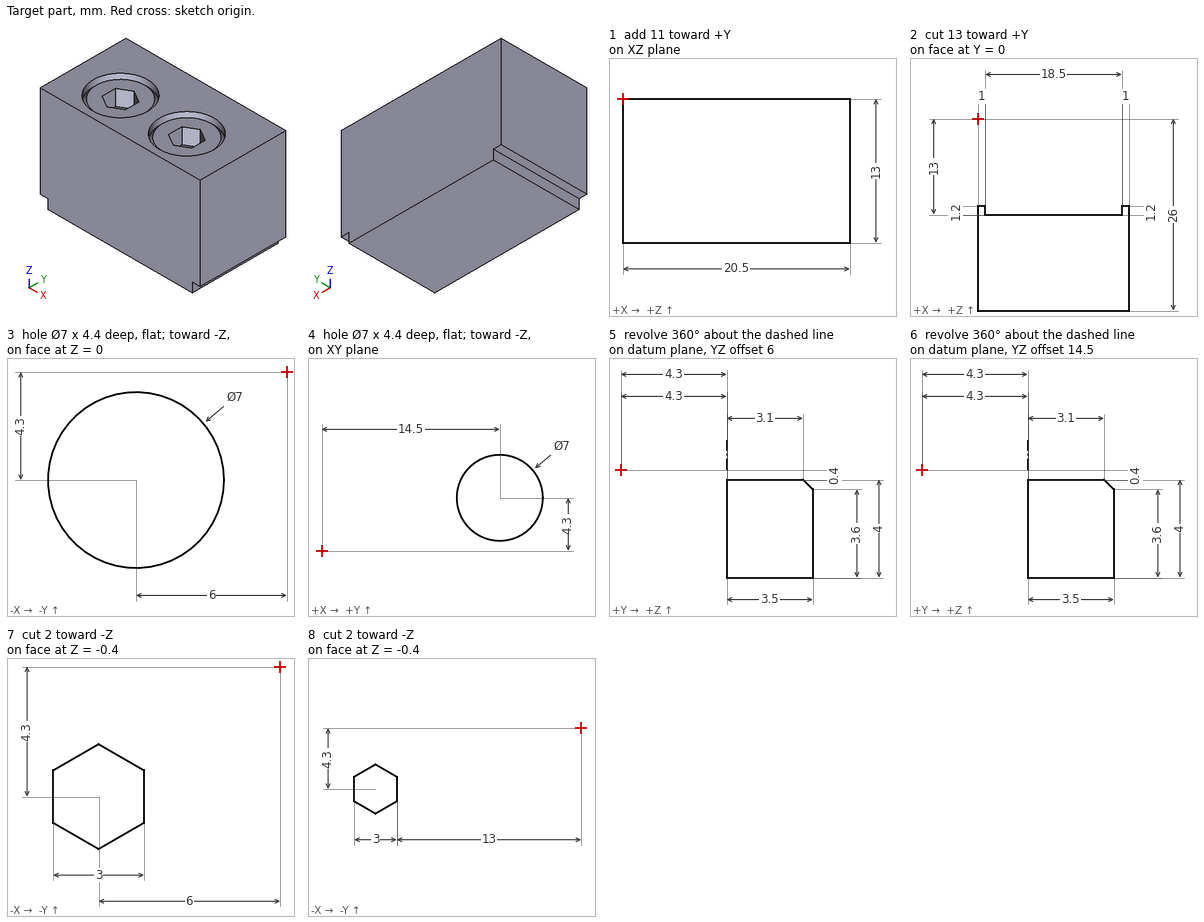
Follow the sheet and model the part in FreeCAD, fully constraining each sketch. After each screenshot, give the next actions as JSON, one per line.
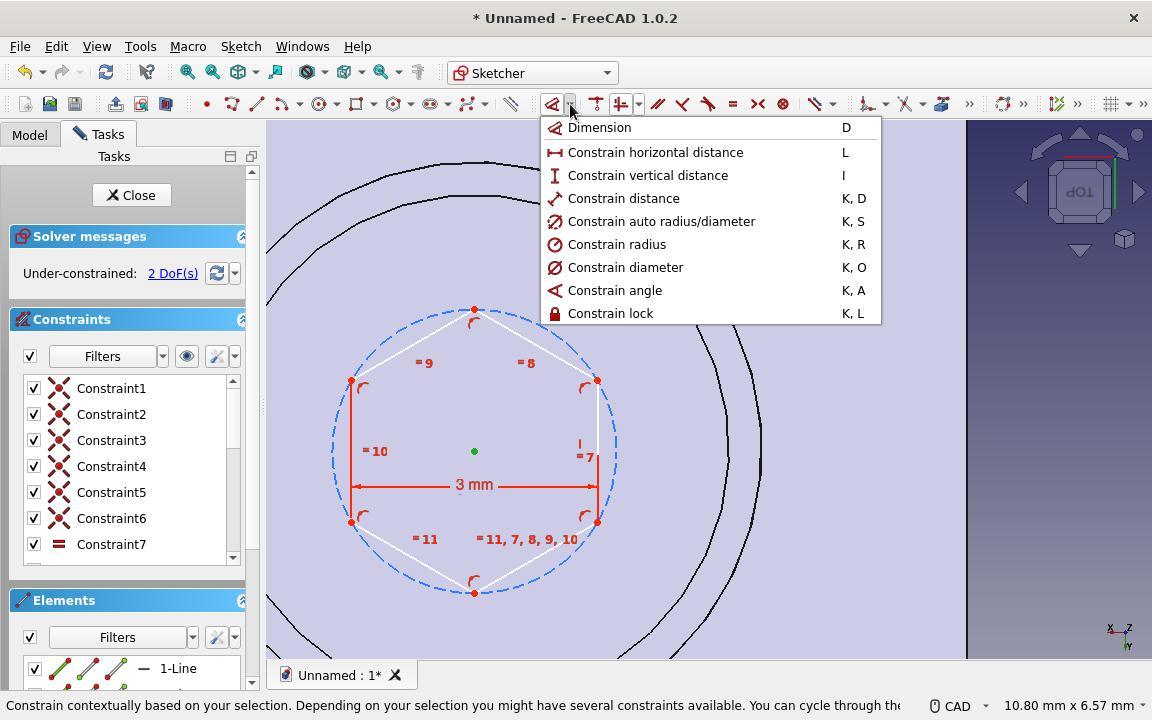
{"action": "left_click", "coordinate": [711, 152]}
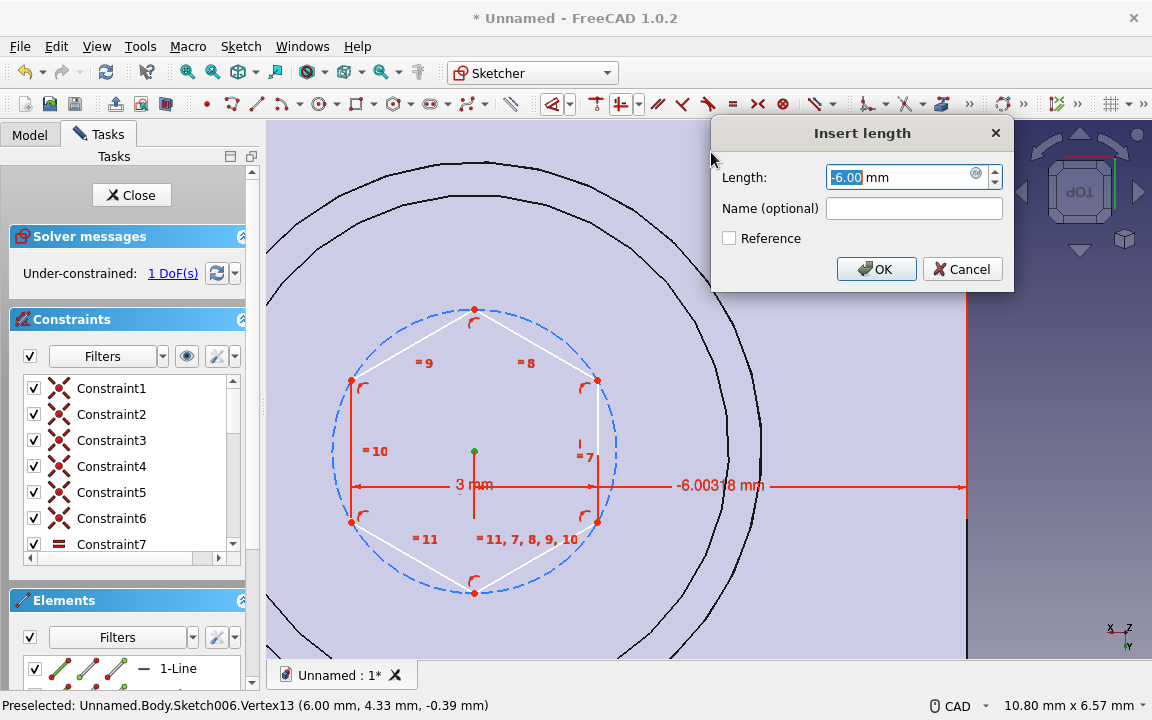
{"action": "type", "text": "-6"}
{"action": "key", "text": "Return"}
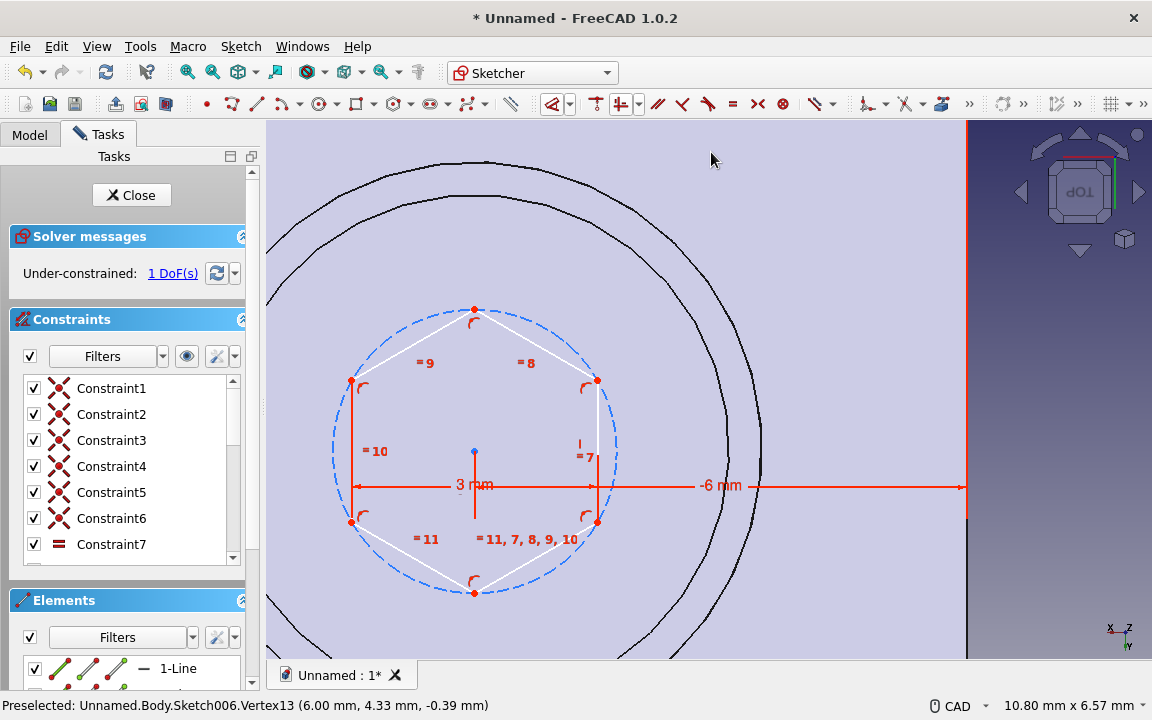
{"action": "left_click", "coordinate": [475, 451]}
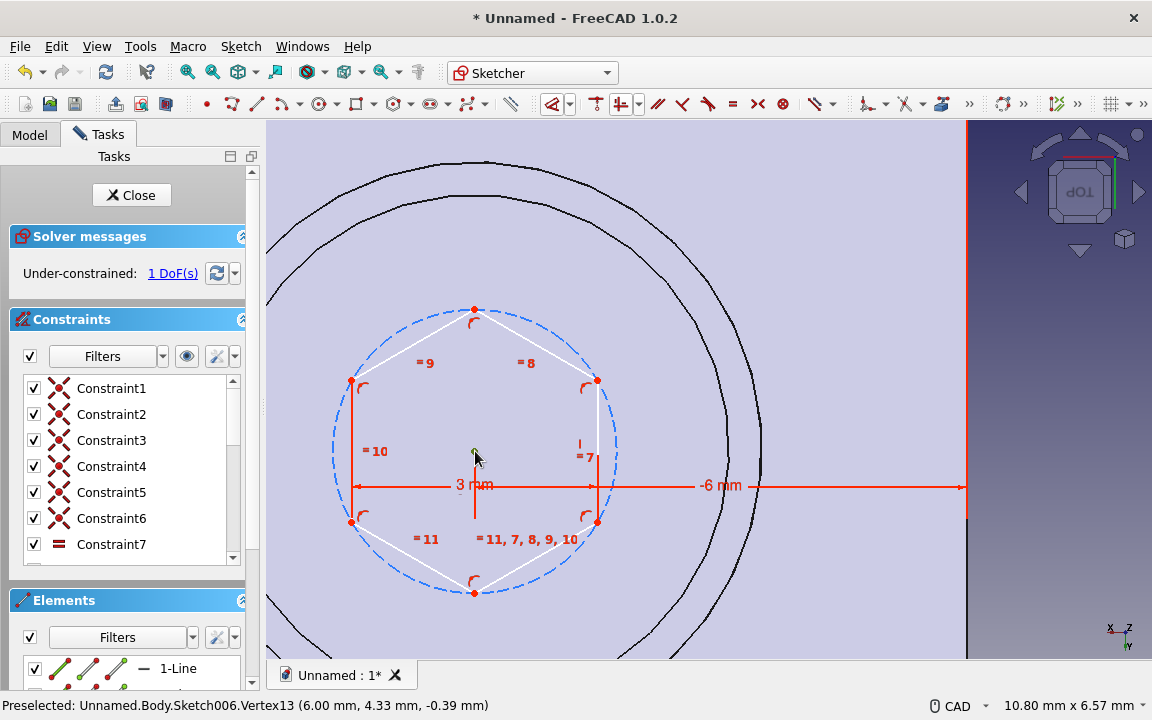
{"action": "key", "text": "i"}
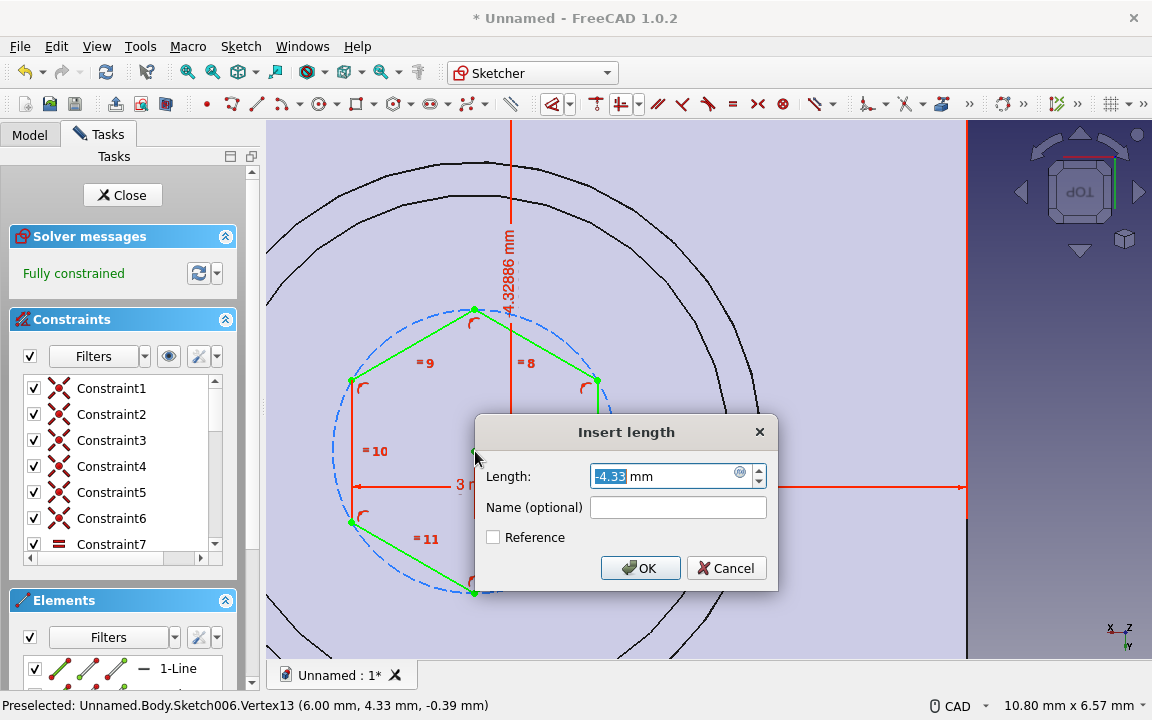
{"action": "type", "text": "-4.3"}
{"action": "key", "text": "Return"}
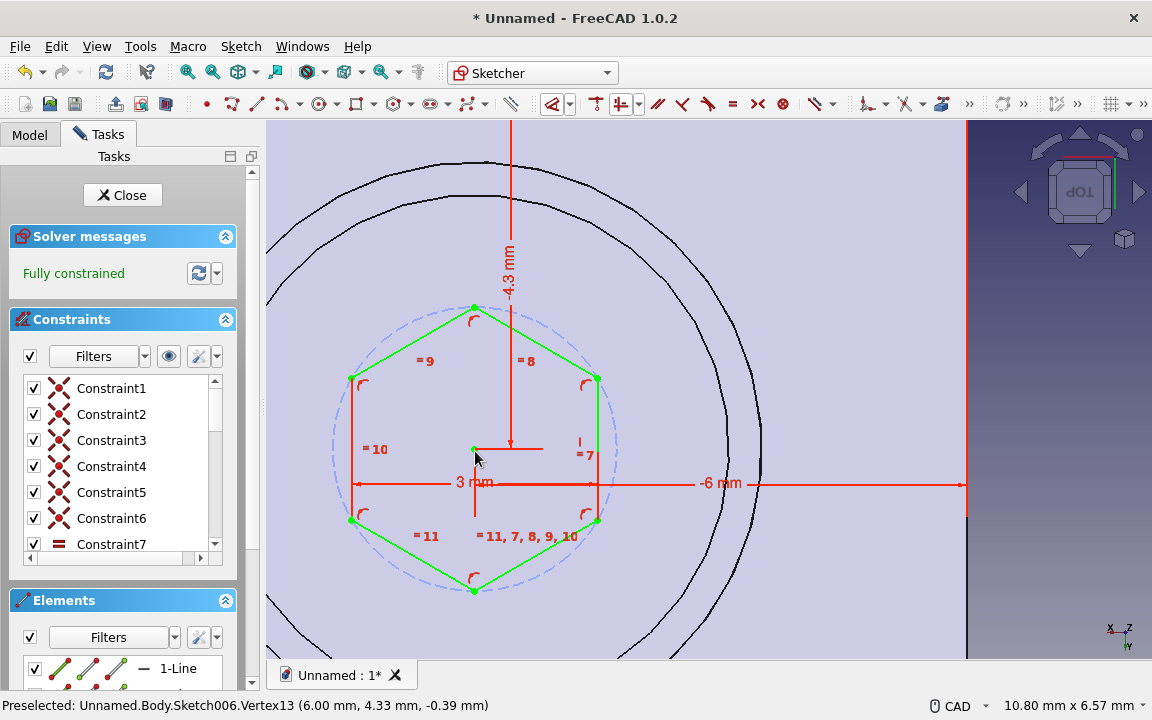
{"action": "left_click", "coordinate": [123, 195]}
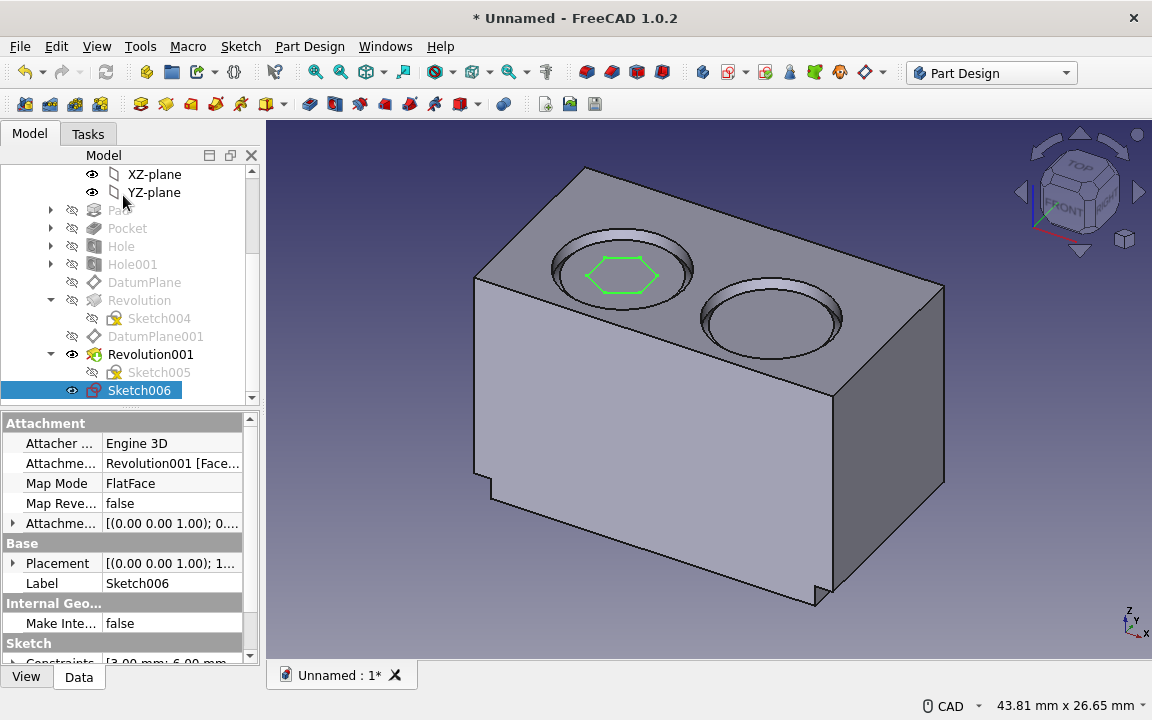
{"action": "left_click", "coordinate": [310, 104]}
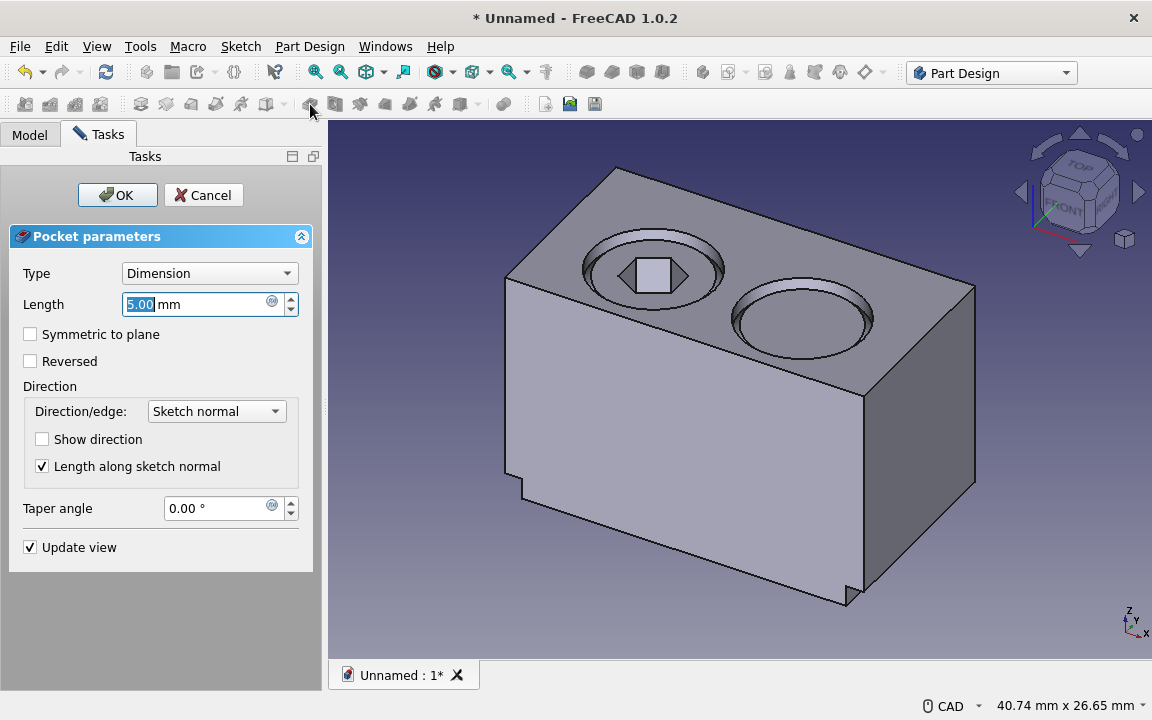
{"action": "type", "text": "2"}
{"action": "key", "text": "Tab"}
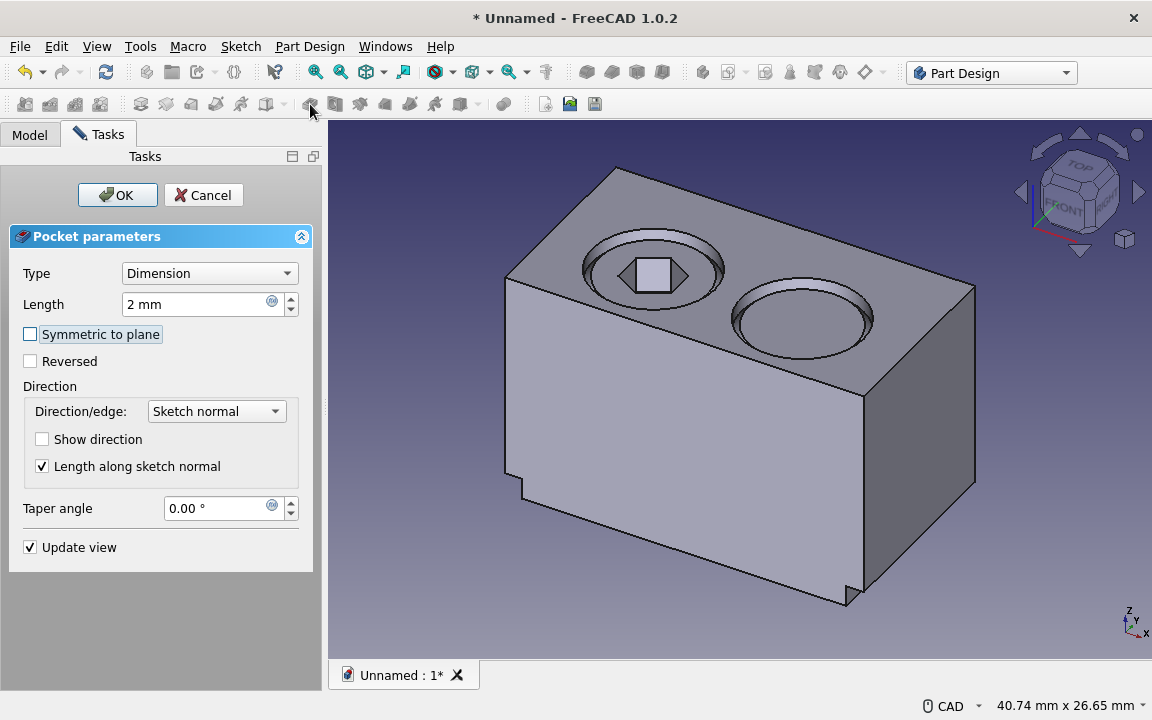
{"action": "left_click", "coordinate": [118, 195]}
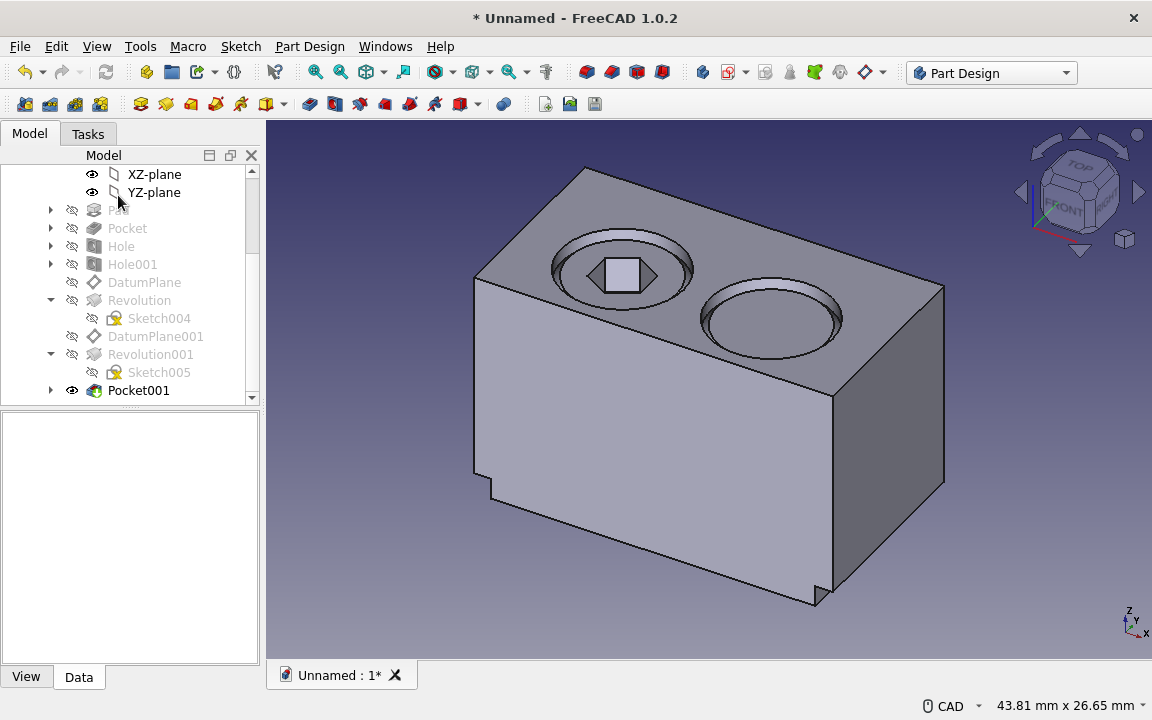
{"action": "left_click", "coordinate": [771, 324]}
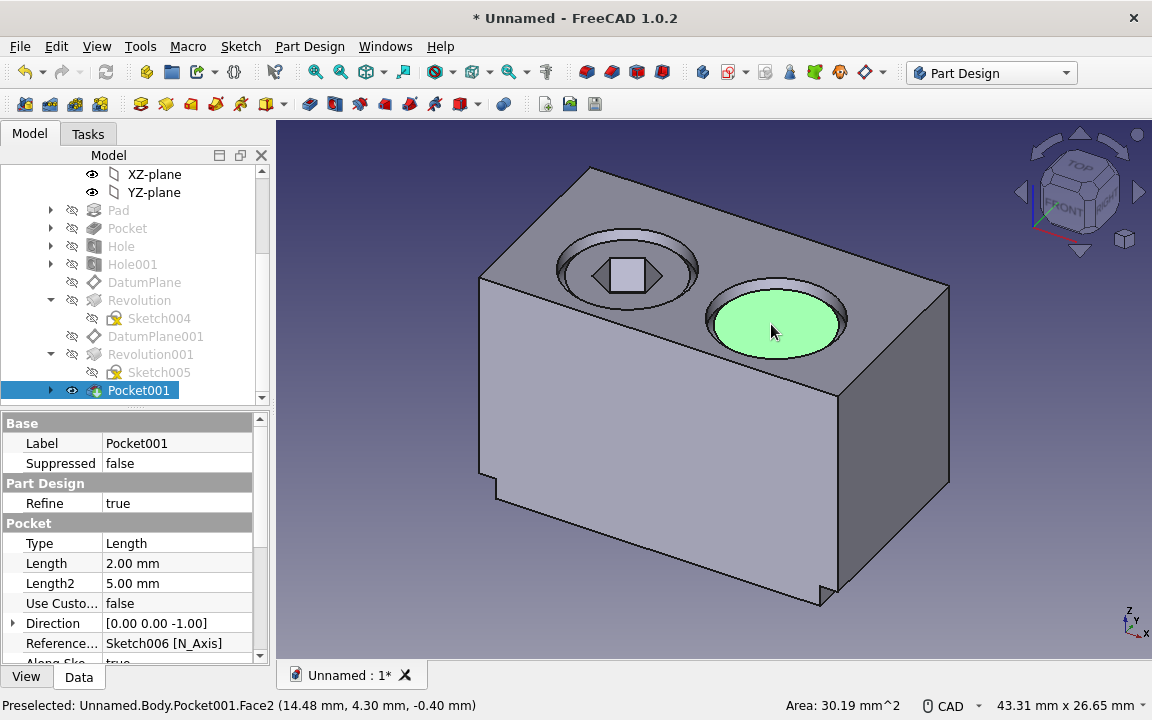
{"action": "left_click", "coordinate": [728, 72]}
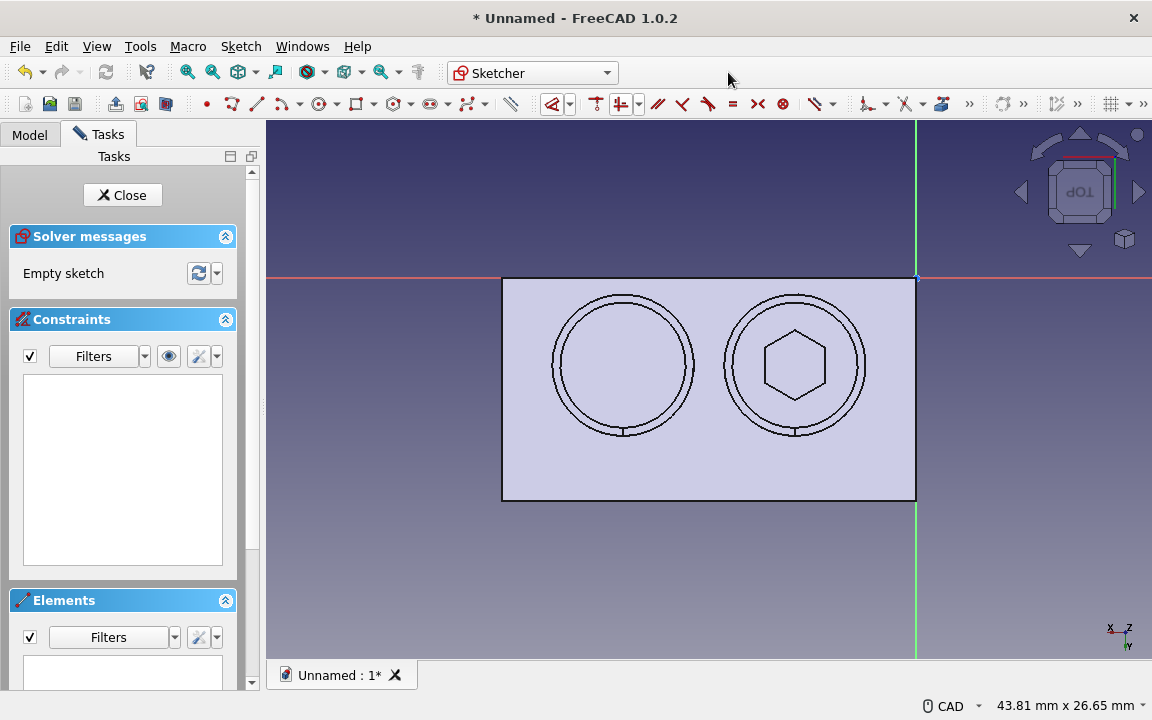
{"action": "left_click", "coordinate": [166, 104]}